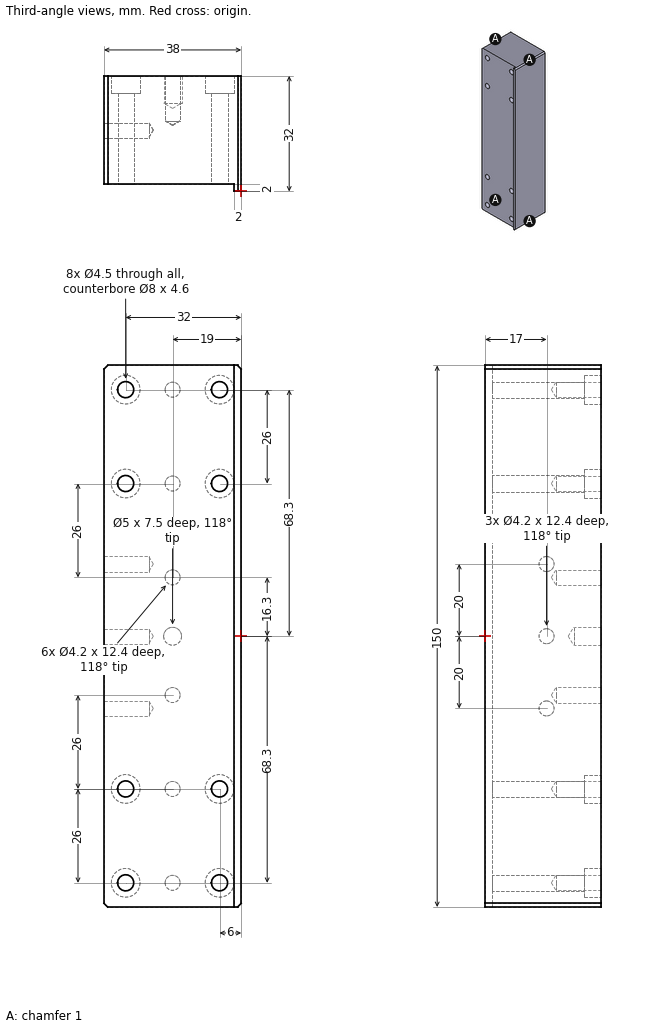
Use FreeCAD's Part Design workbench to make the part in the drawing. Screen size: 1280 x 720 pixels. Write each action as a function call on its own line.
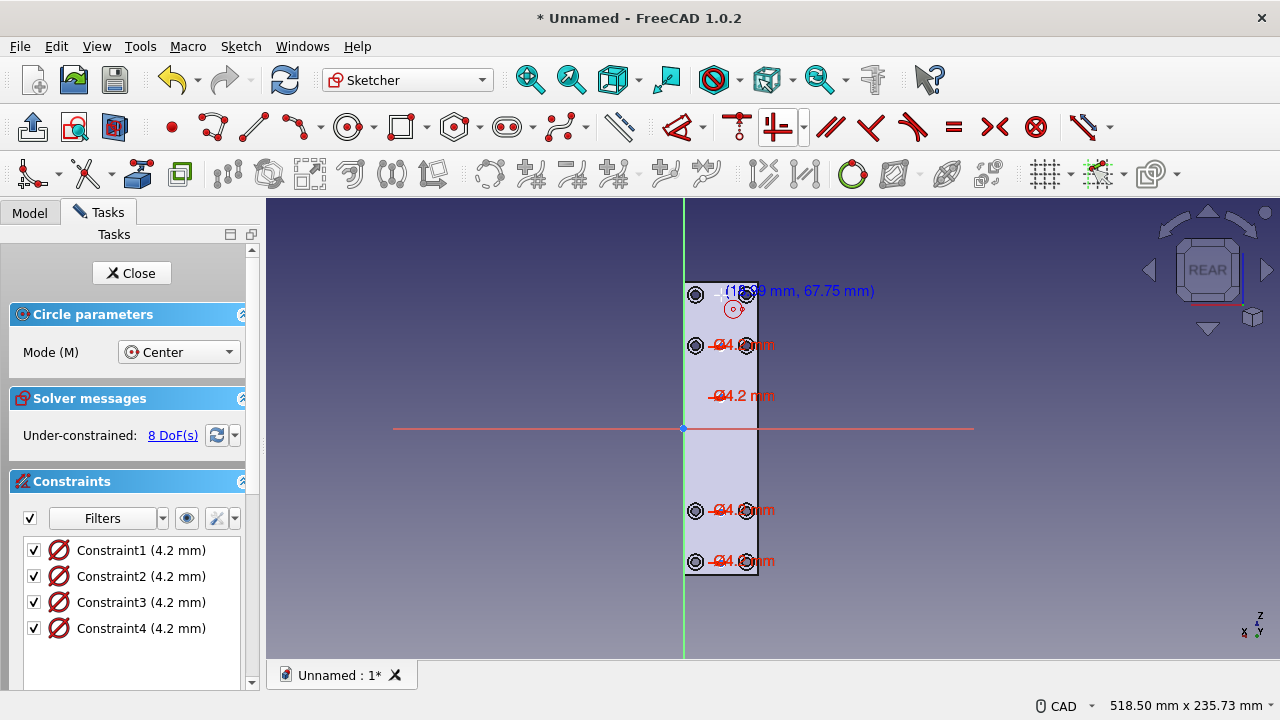
click(721, 295)
move(724, 292)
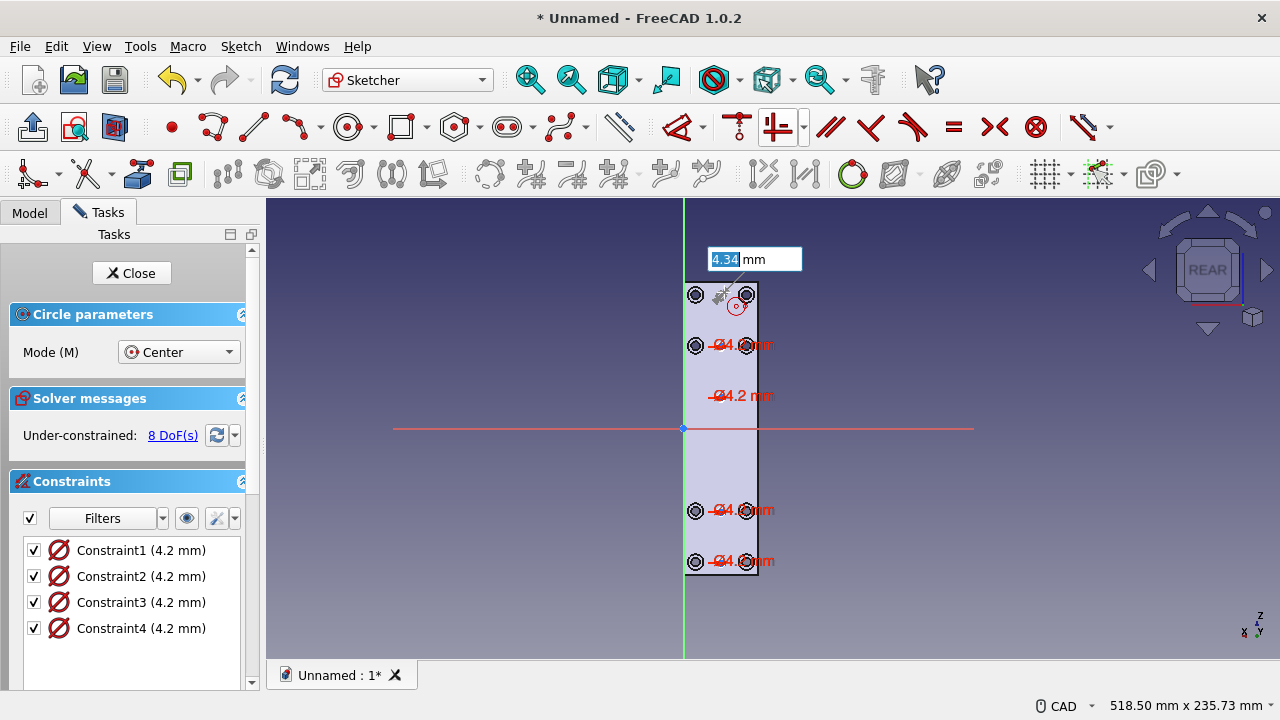
text(4.2)
key(Return)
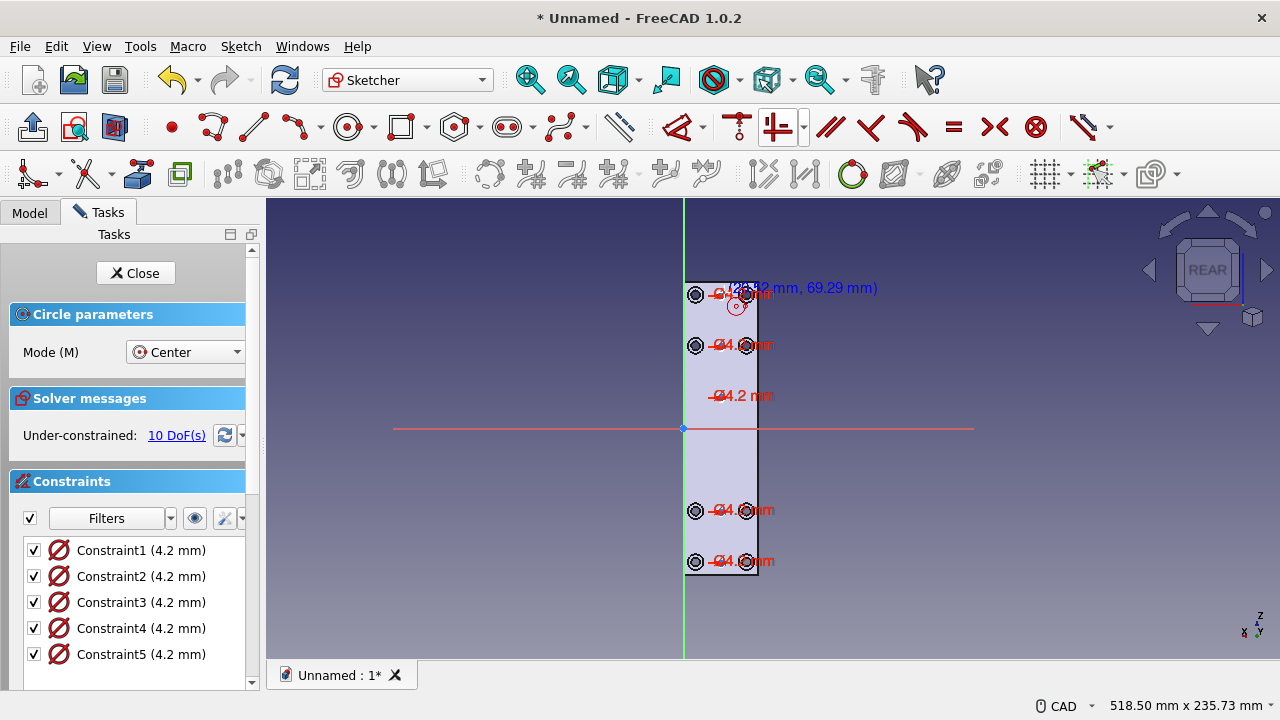
scroll(721, 460, up, 9)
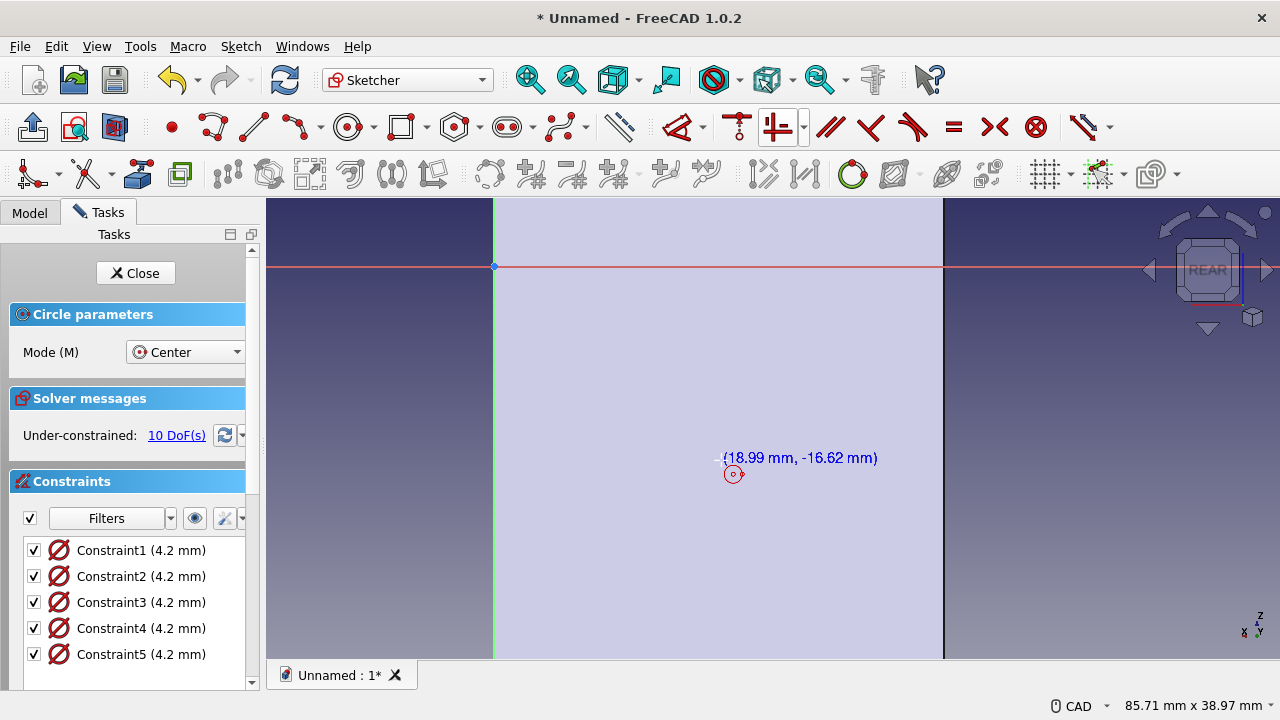
scroll(721, 461, down, 9)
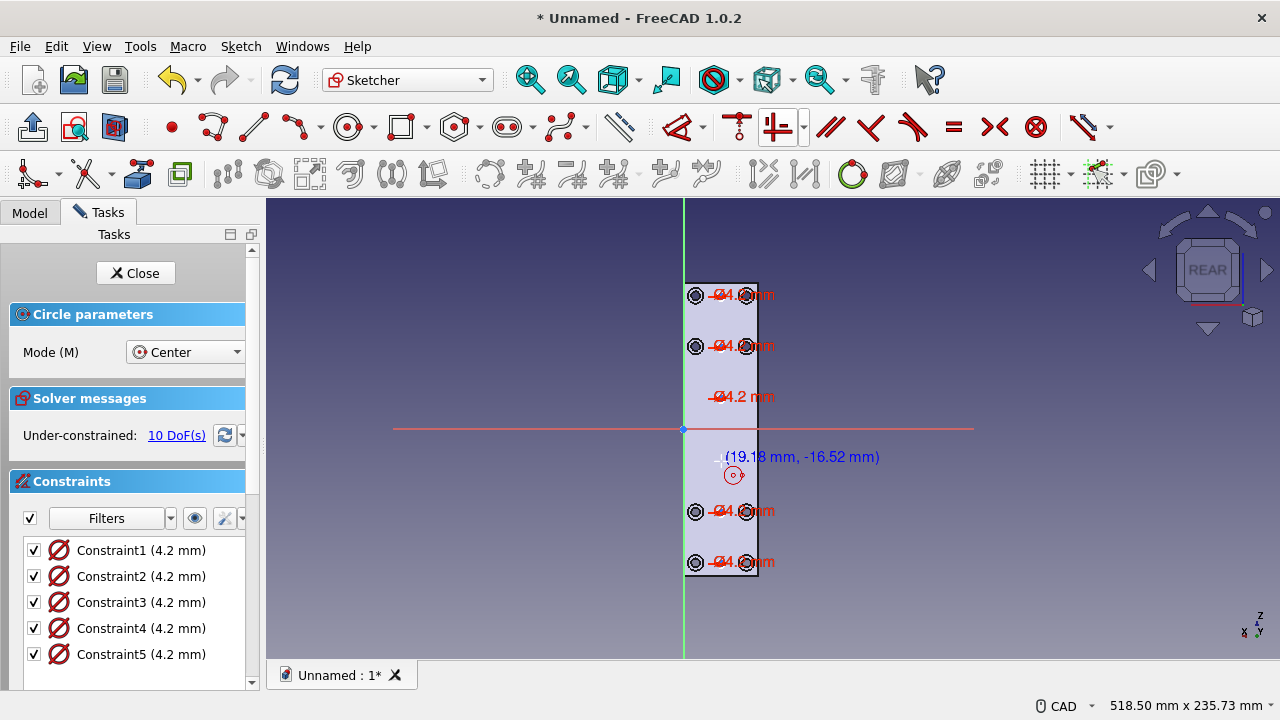
click(721, 461)
move(724, 458)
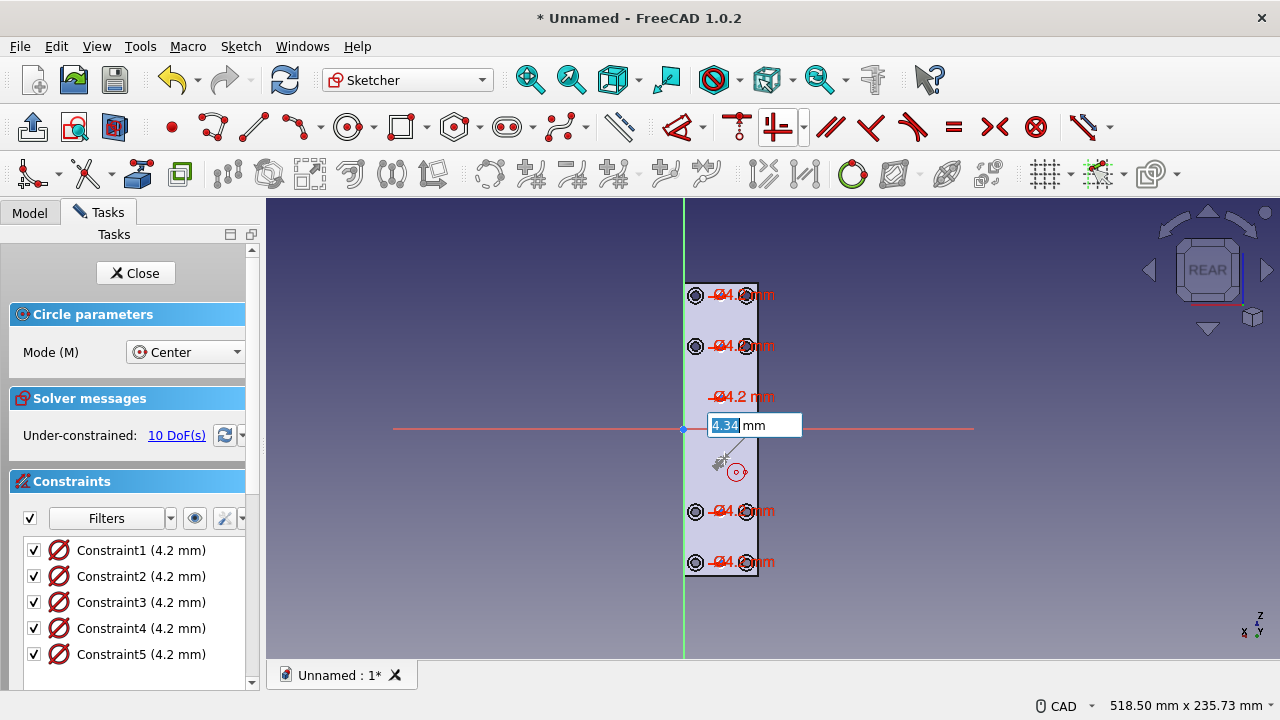
text(4.2)
key(Return)
key(Escape)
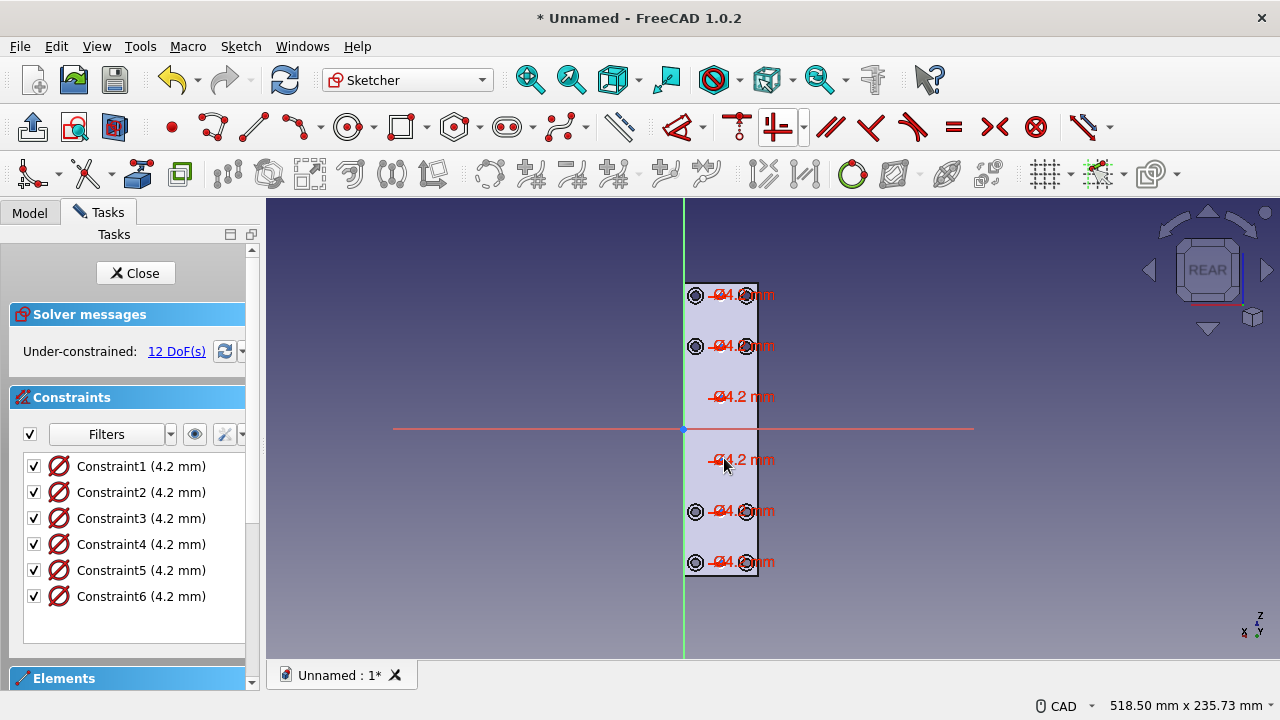
click(676, 128)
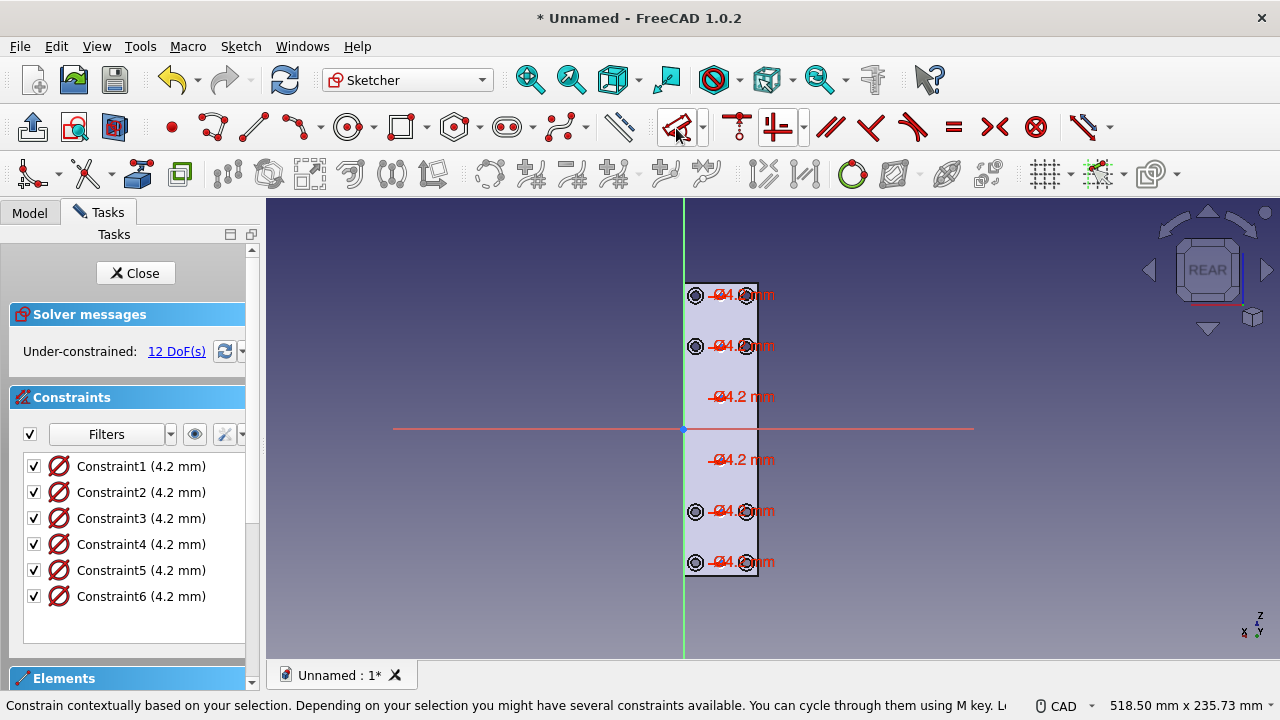
click(721, 399)
click(702, 365)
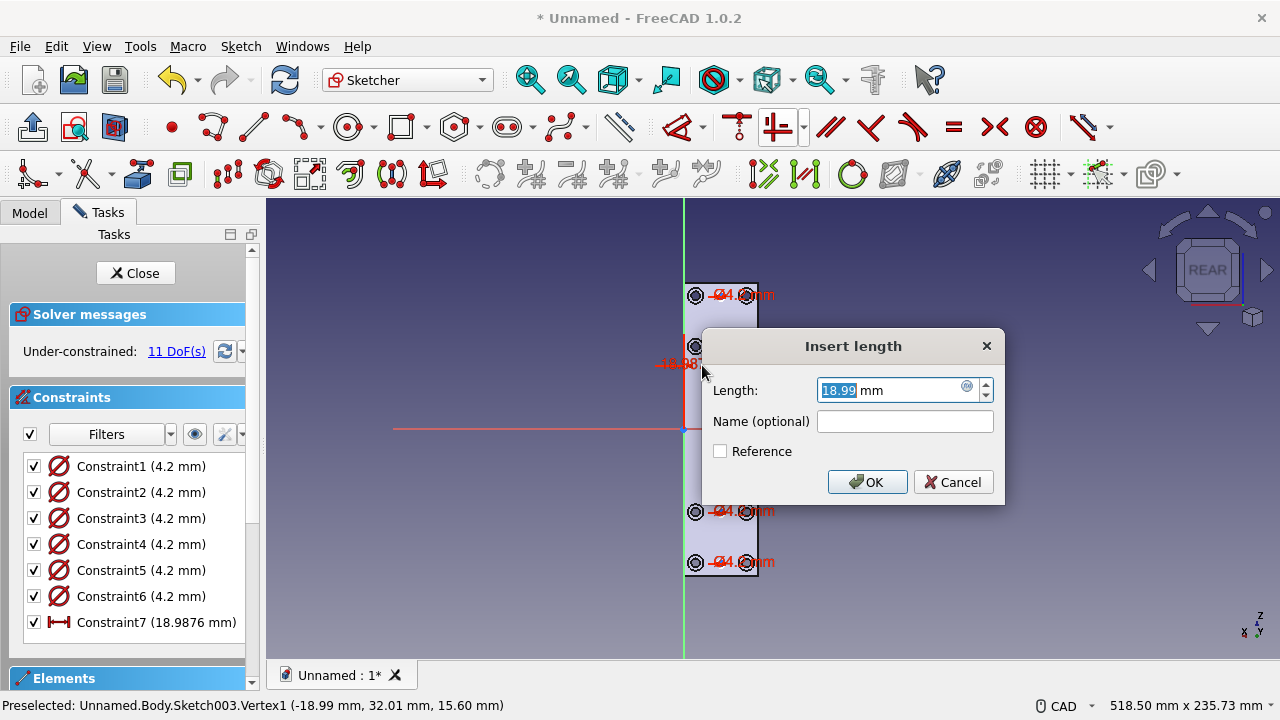
text(19)
key(Return)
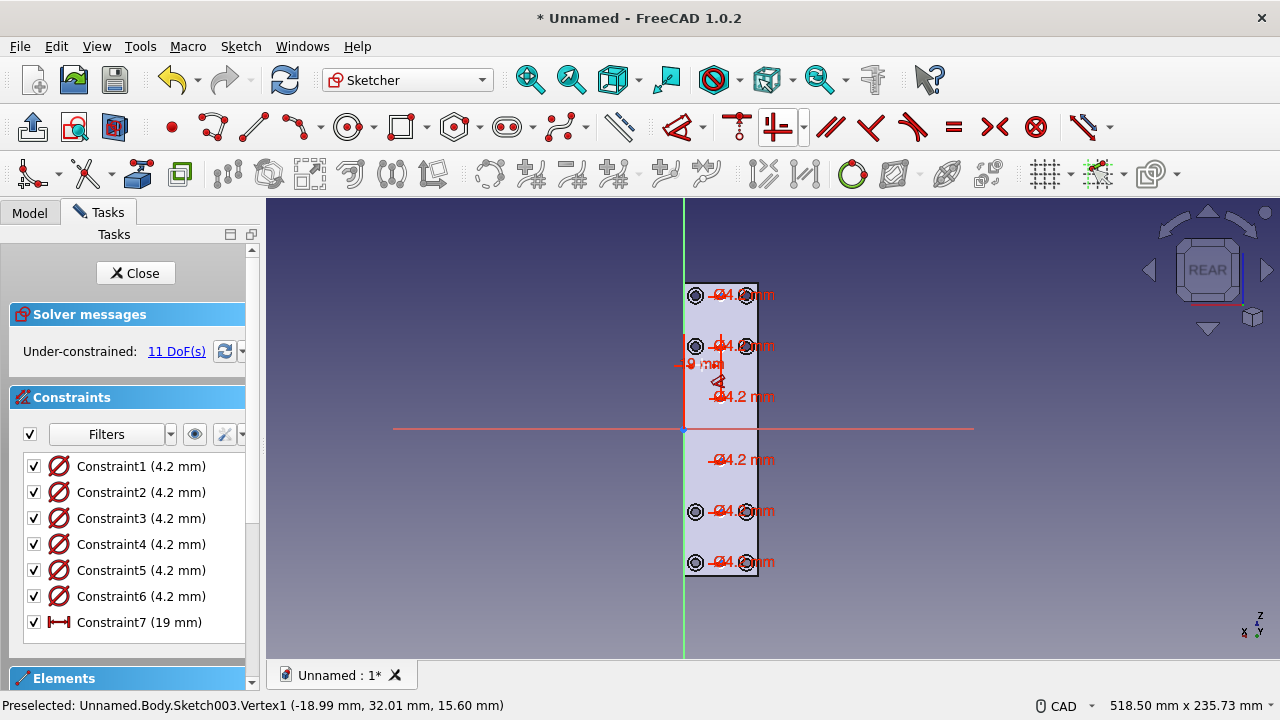
click(721, 564)
click(702, 598)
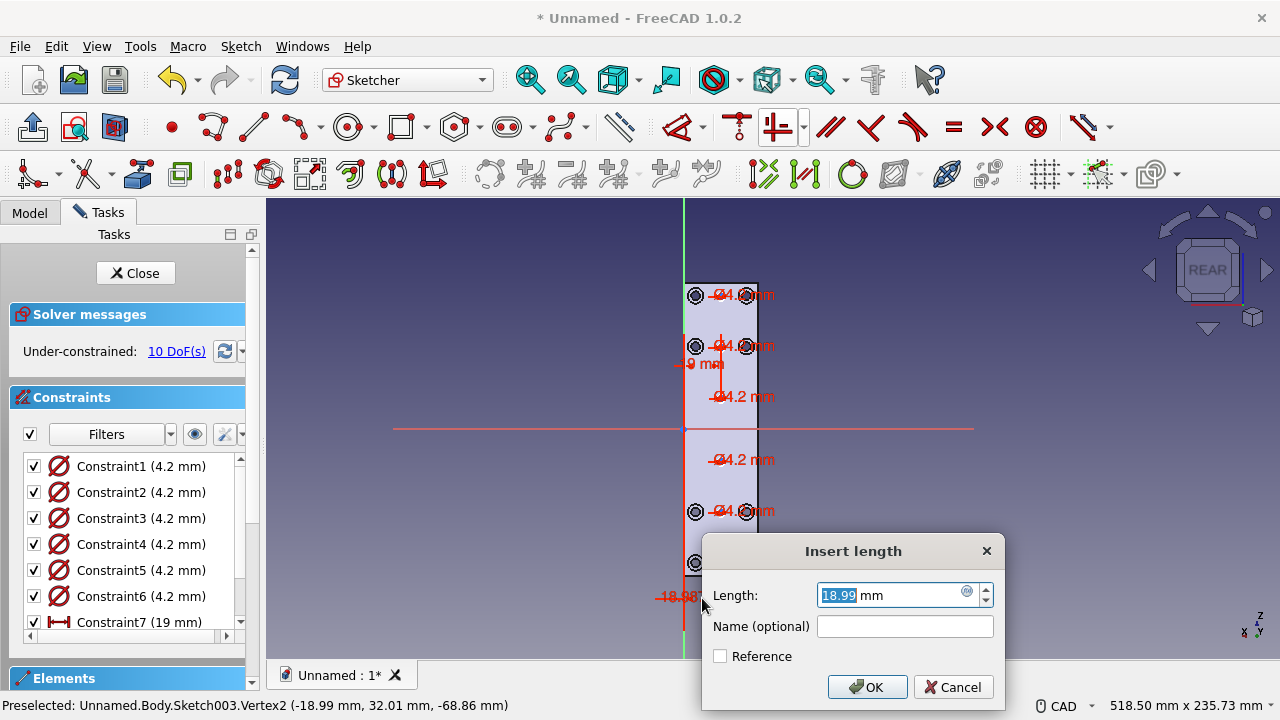
text(19)
key(Return)